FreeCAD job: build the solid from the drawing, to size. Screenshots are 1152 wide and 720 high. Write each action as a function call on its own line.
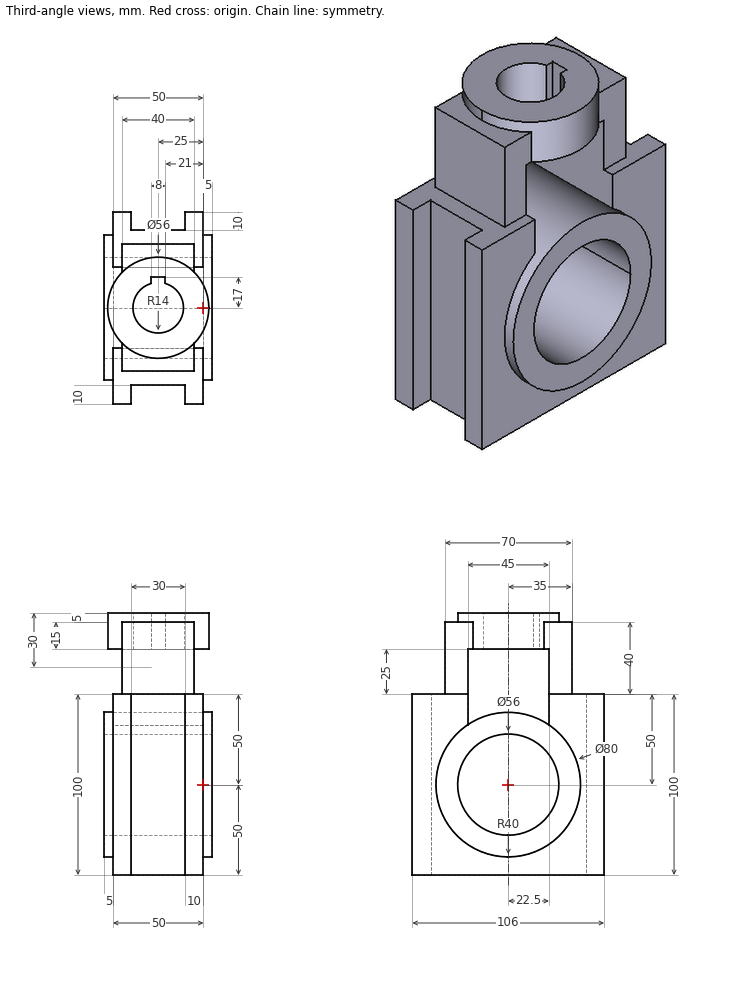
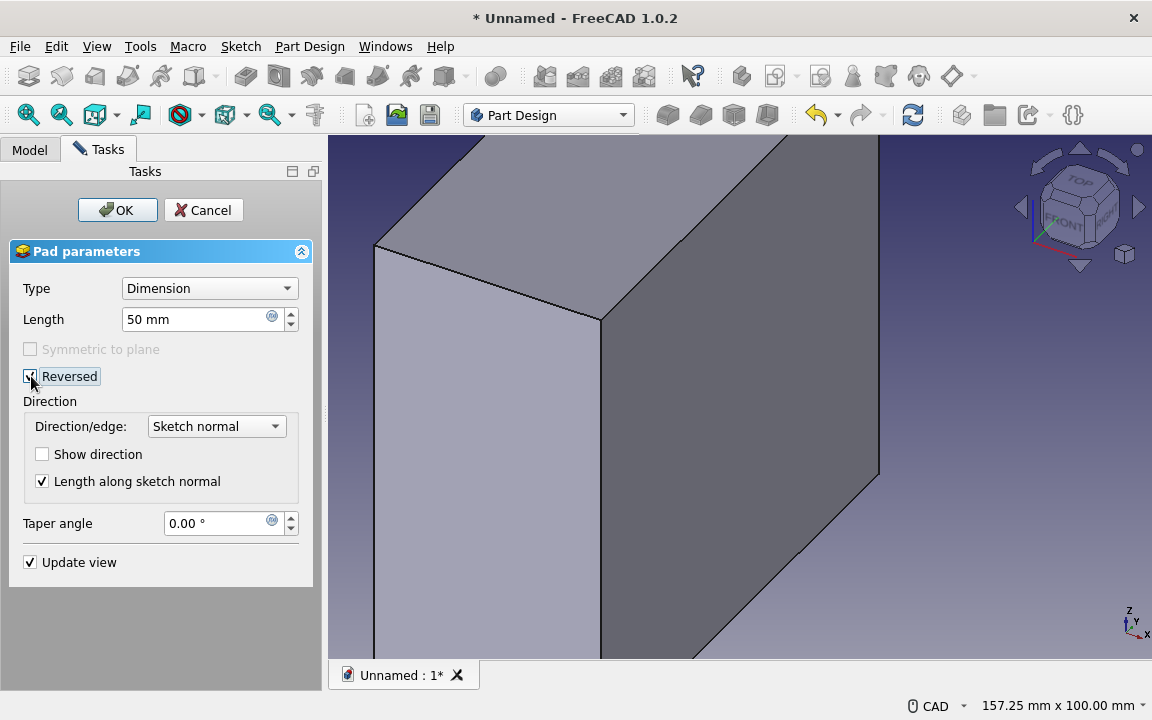
click(118, 210)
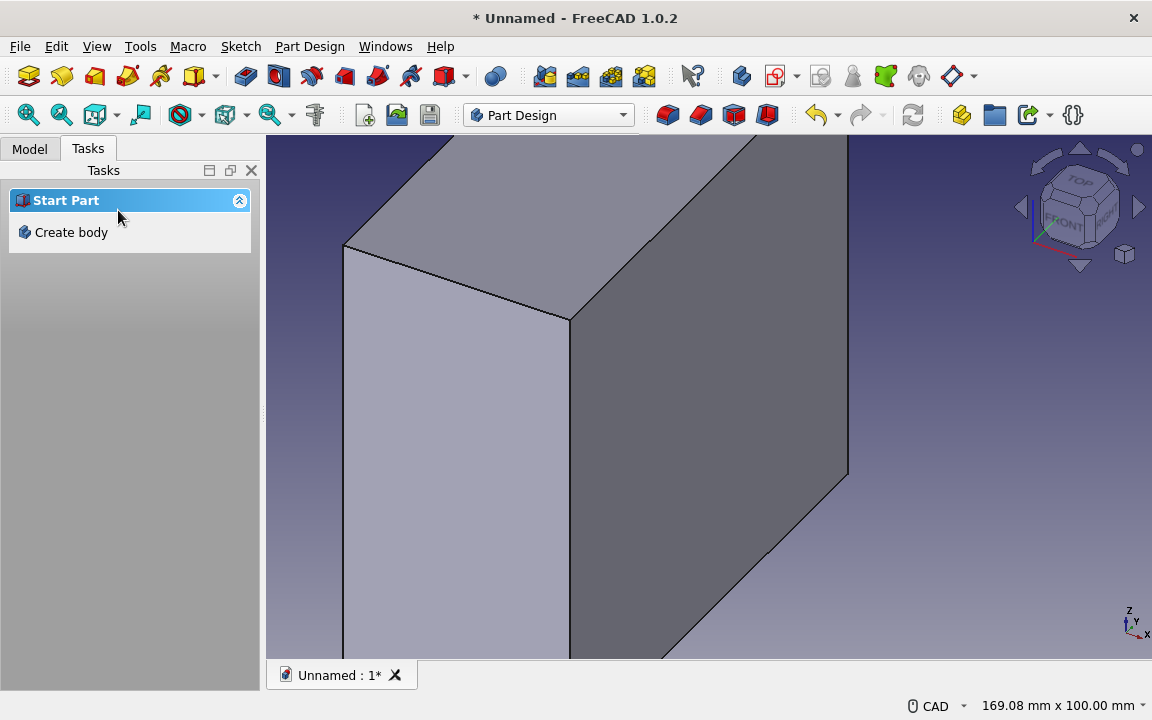
key(v)
key(f)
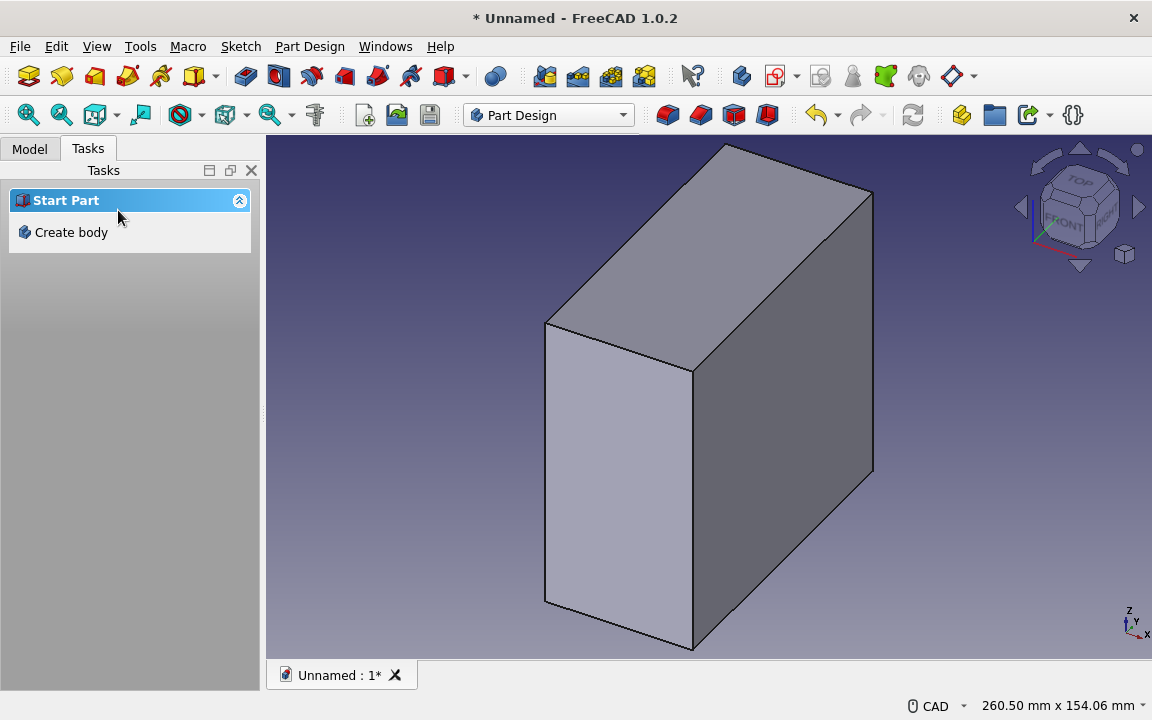
click(783, 420)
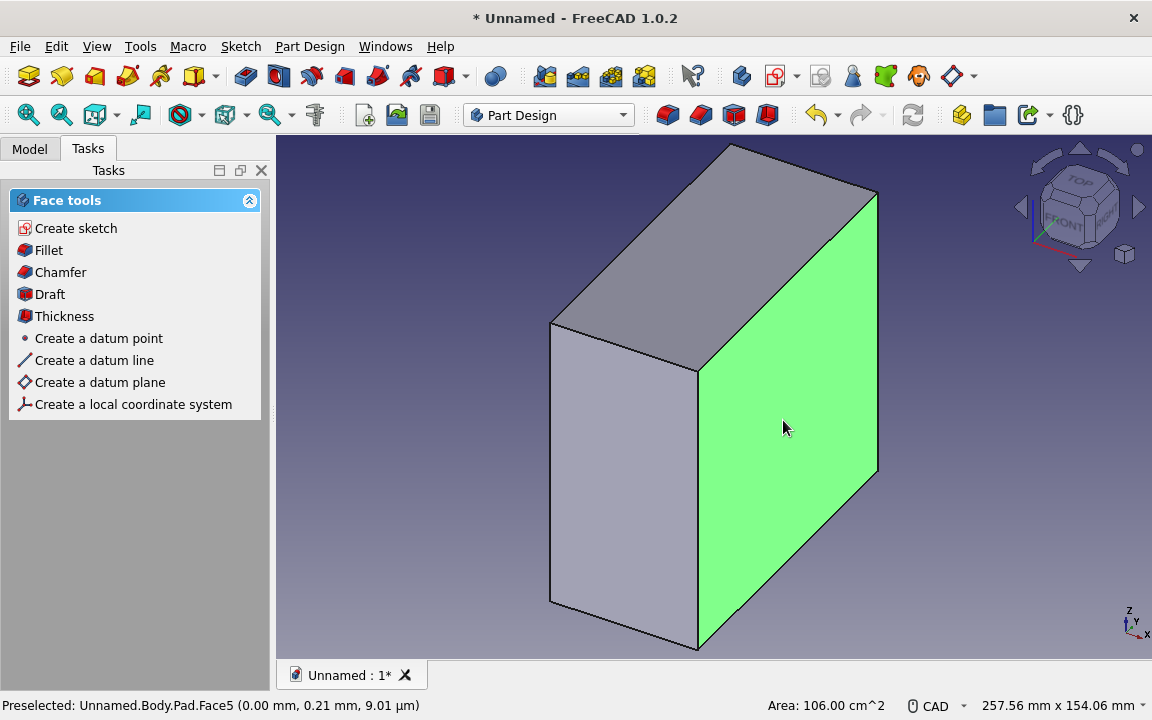
click(774, 76)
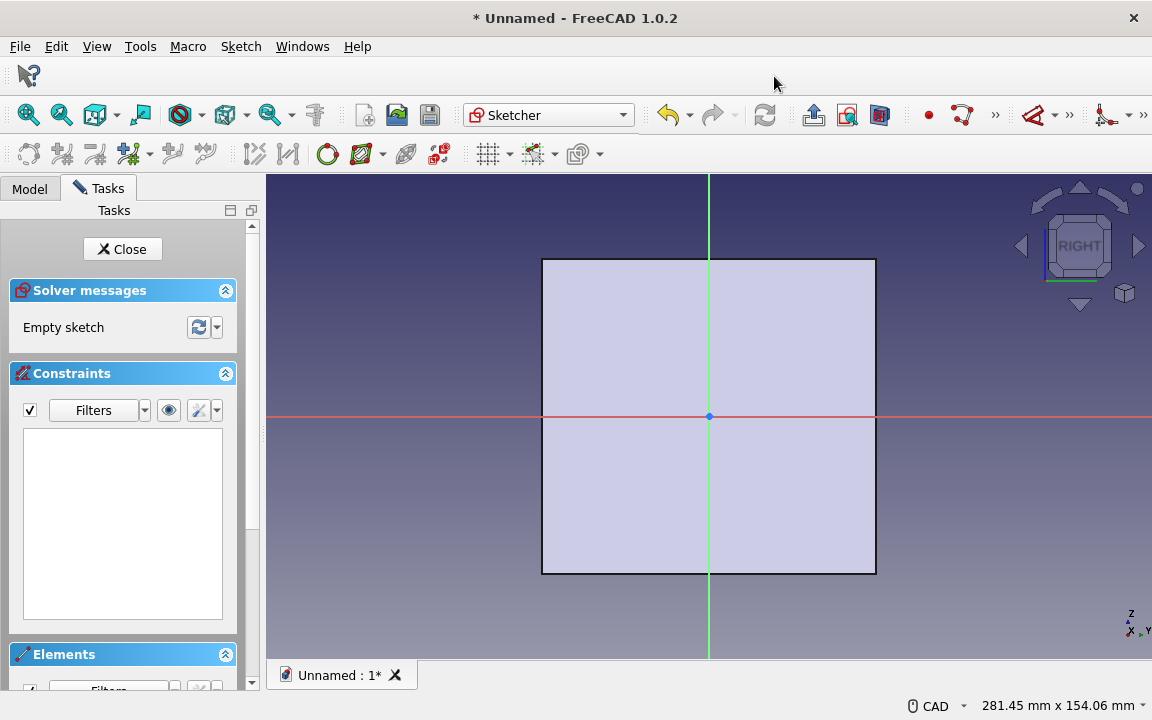
click(962, 116)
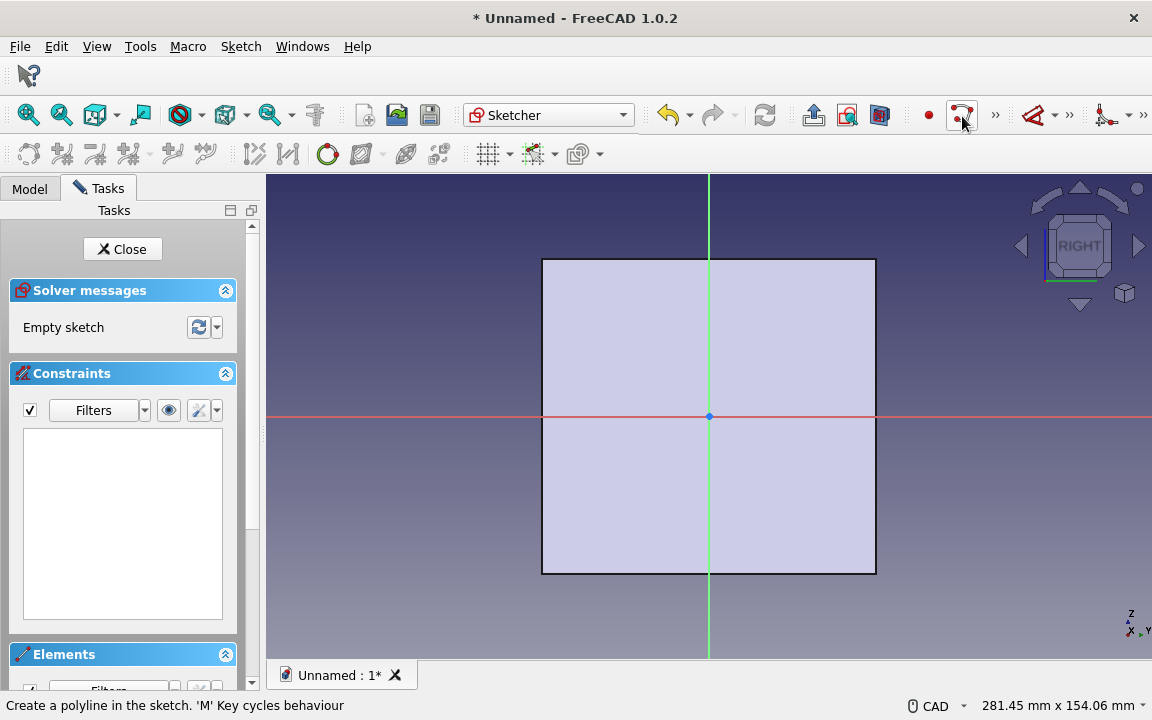
click(780, 312)
click(780, 259)
click(638, 259)
click(638, 312)
right_click(638, 312)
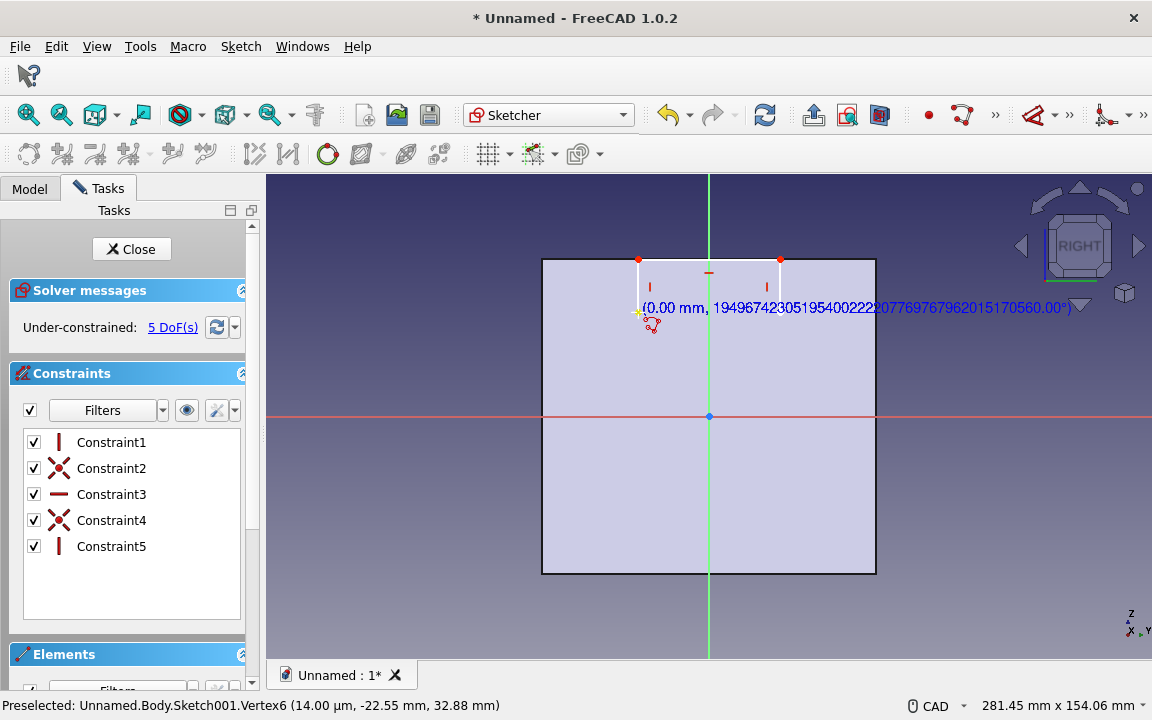
key(g)
key(3)
key(a)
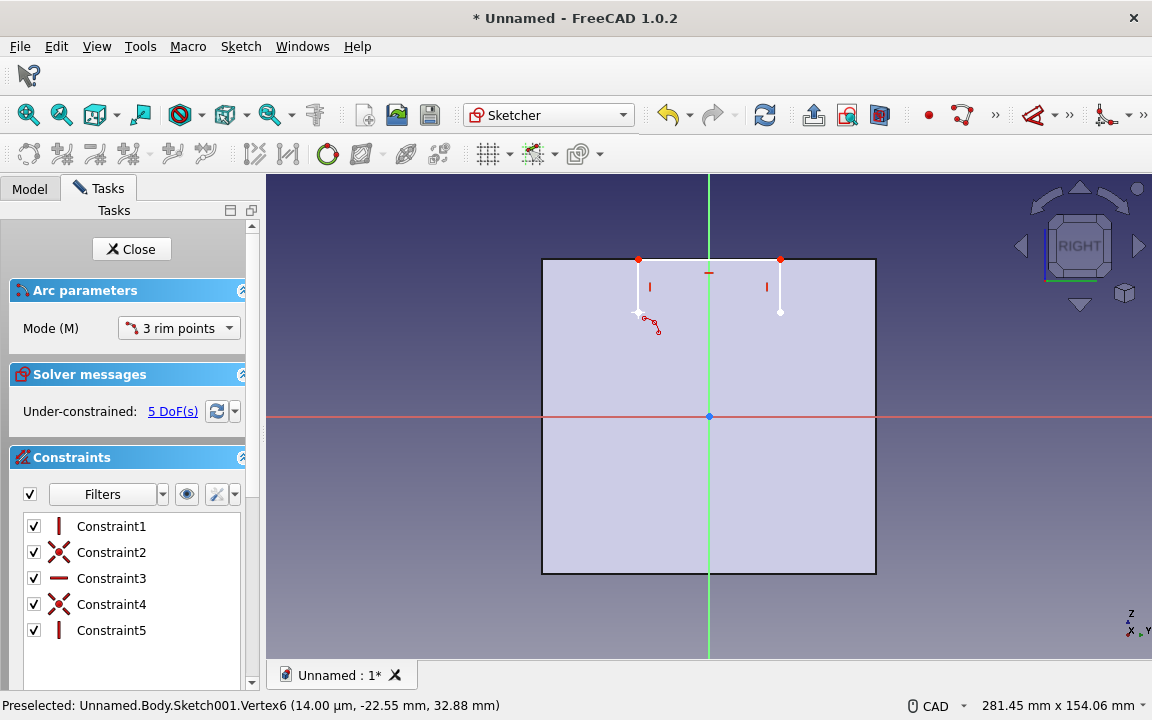
click(638, 313)
click(780, 313)
click(648, 526)
key(Escape)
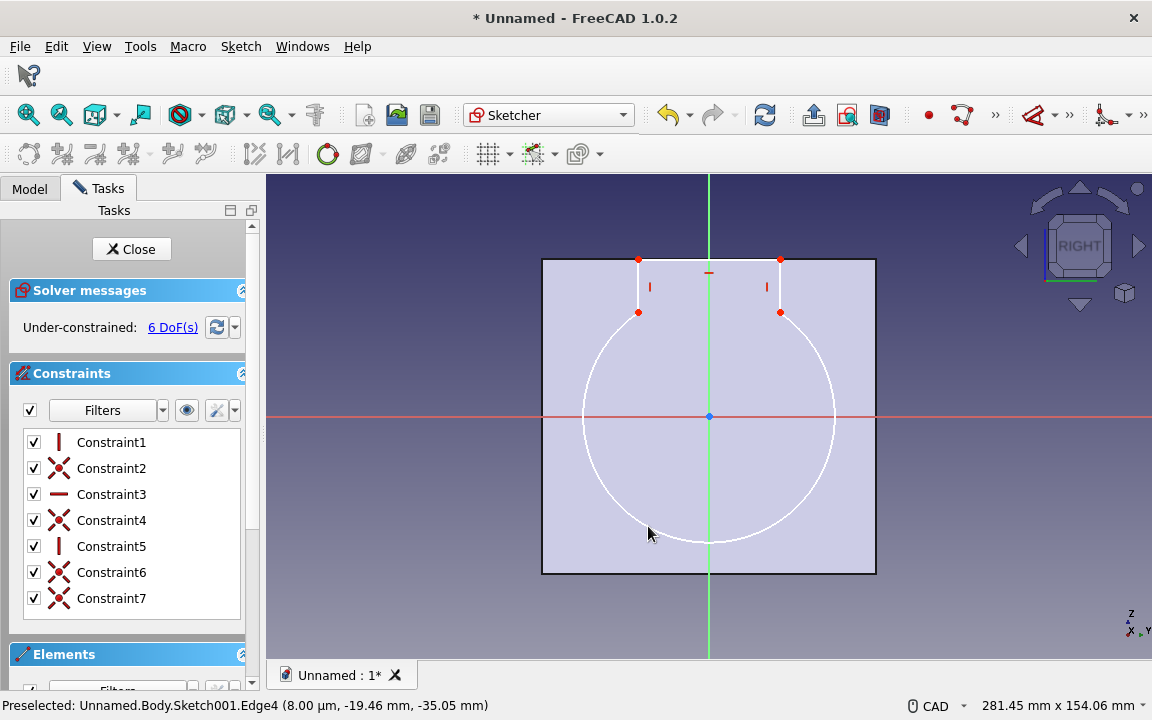
drag(699, 406, 719, 427)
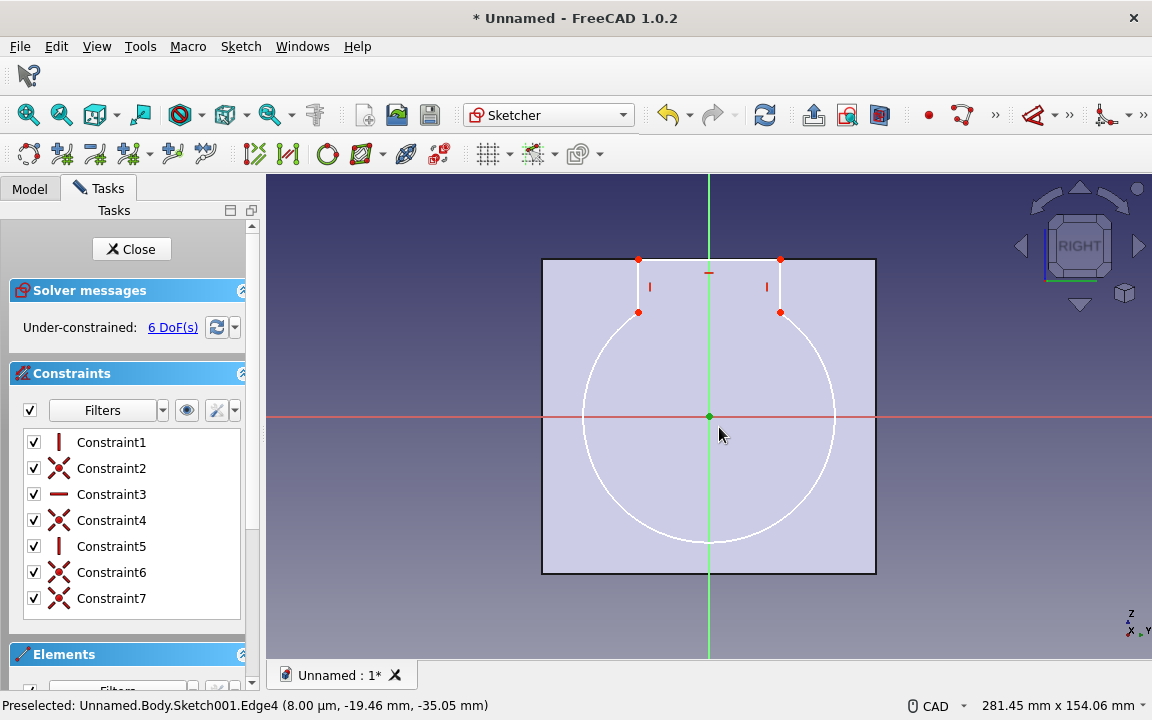
key(c)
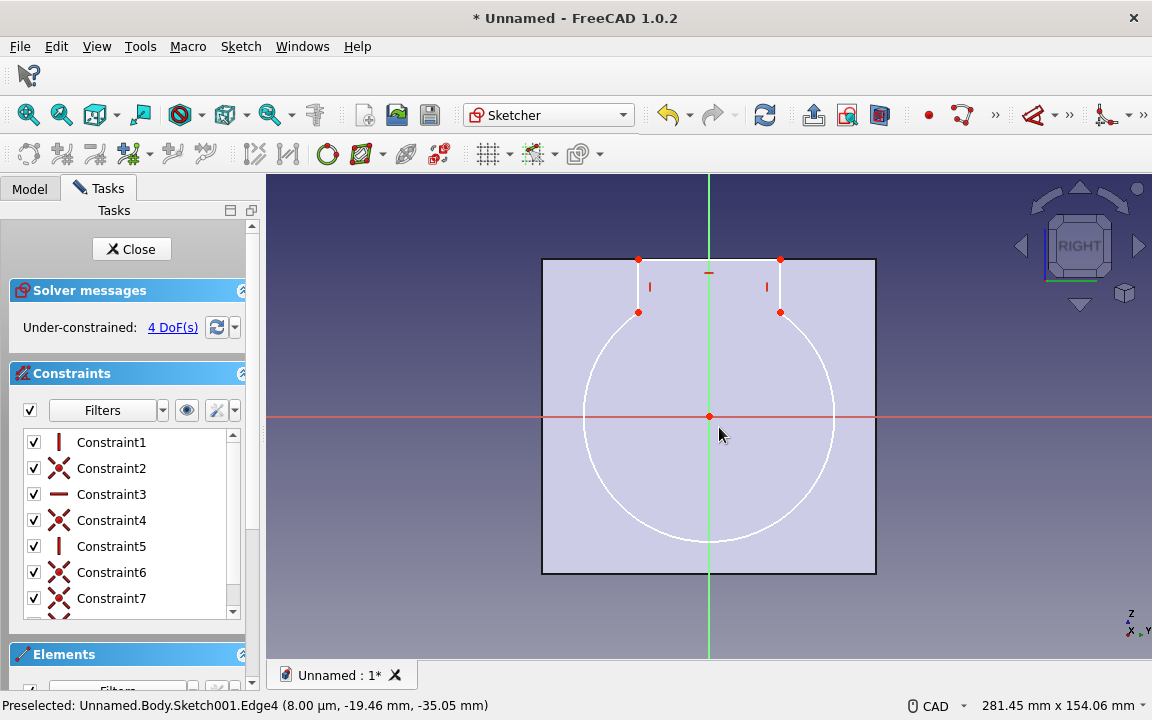
click(1032, 116)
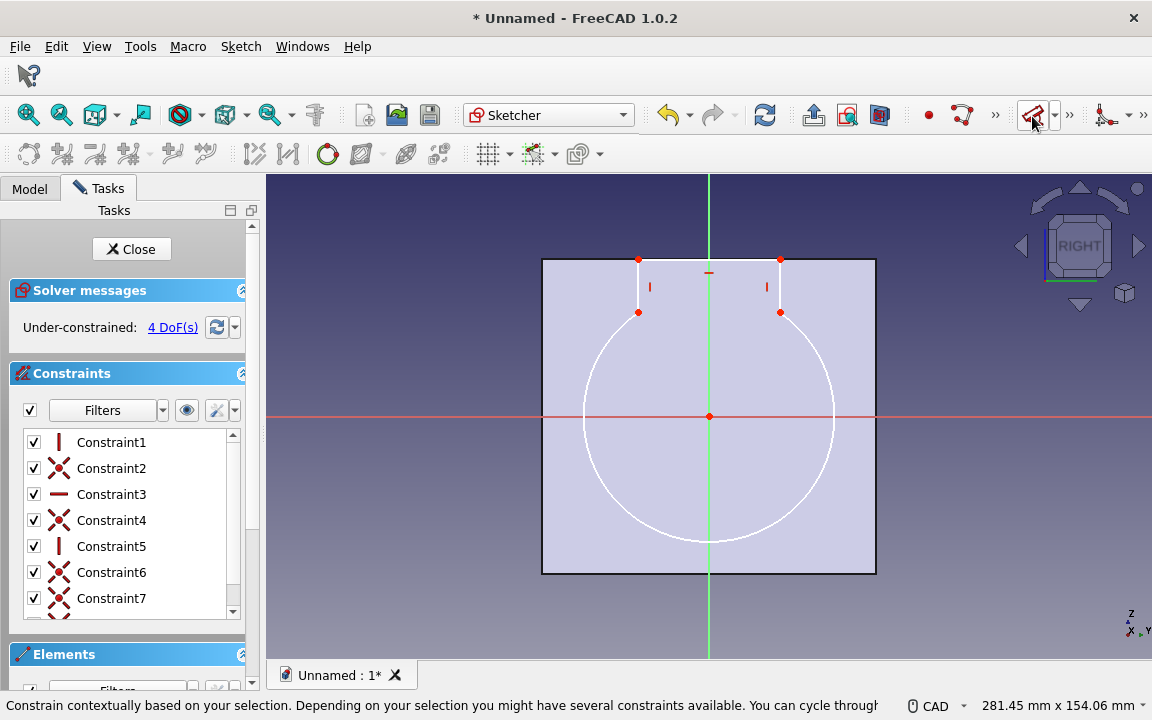
click(602, 483)
click(575, 500)